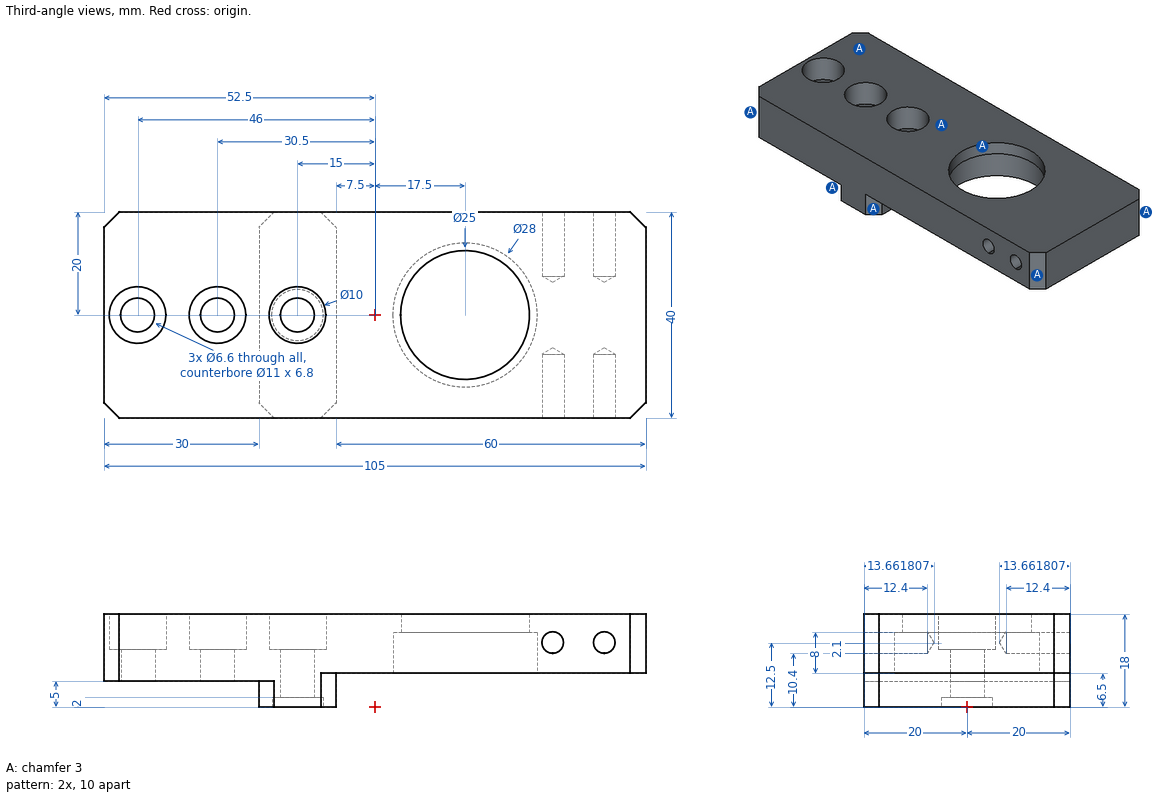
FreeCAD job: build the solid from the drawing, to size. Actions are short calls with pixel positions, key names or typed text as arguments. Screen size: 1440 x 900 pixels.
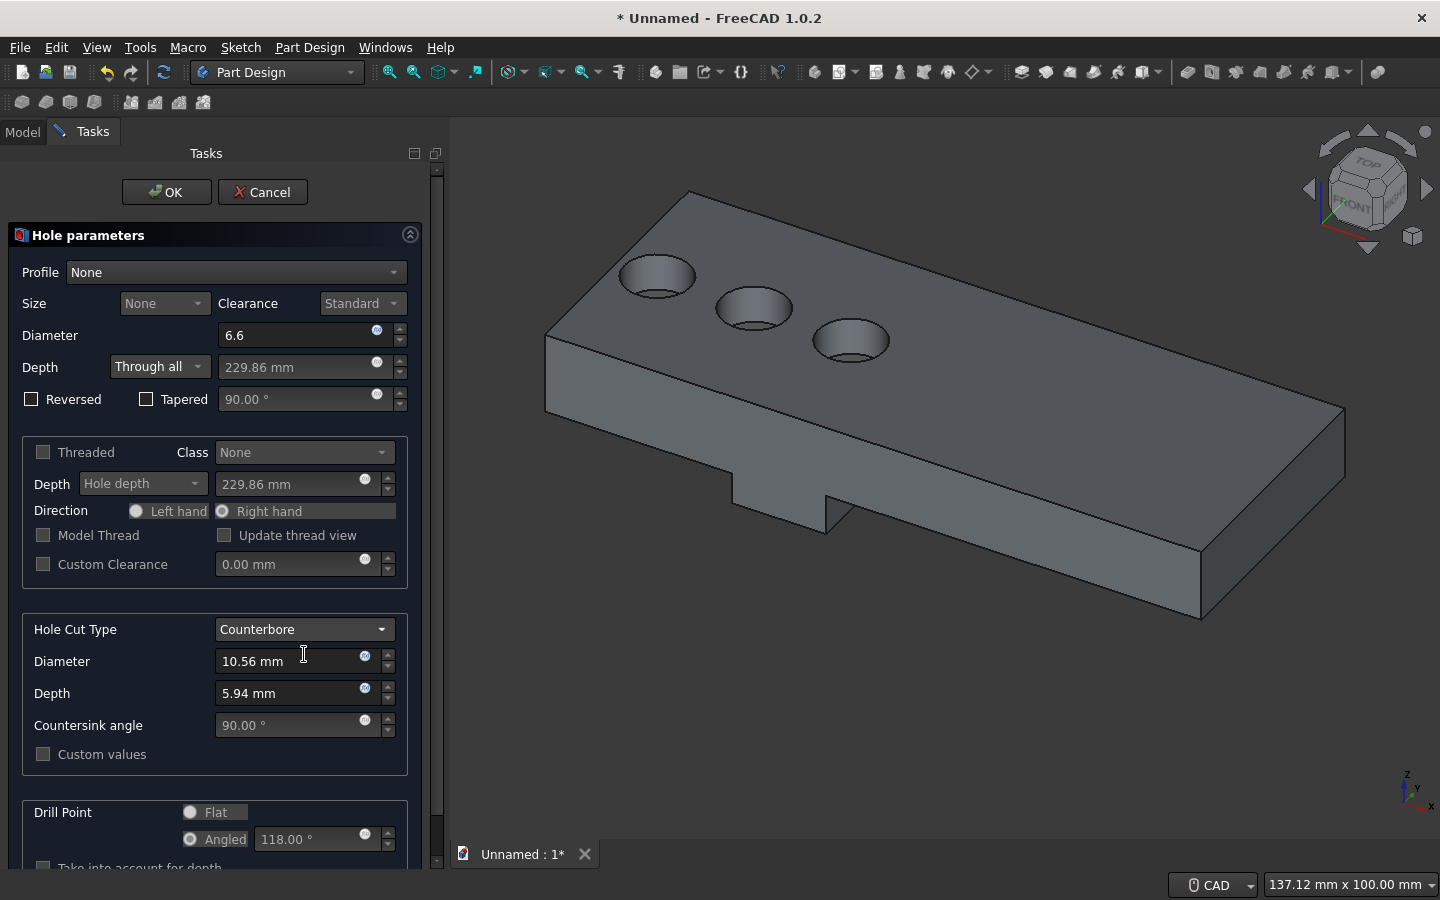
triple_click(298, 661)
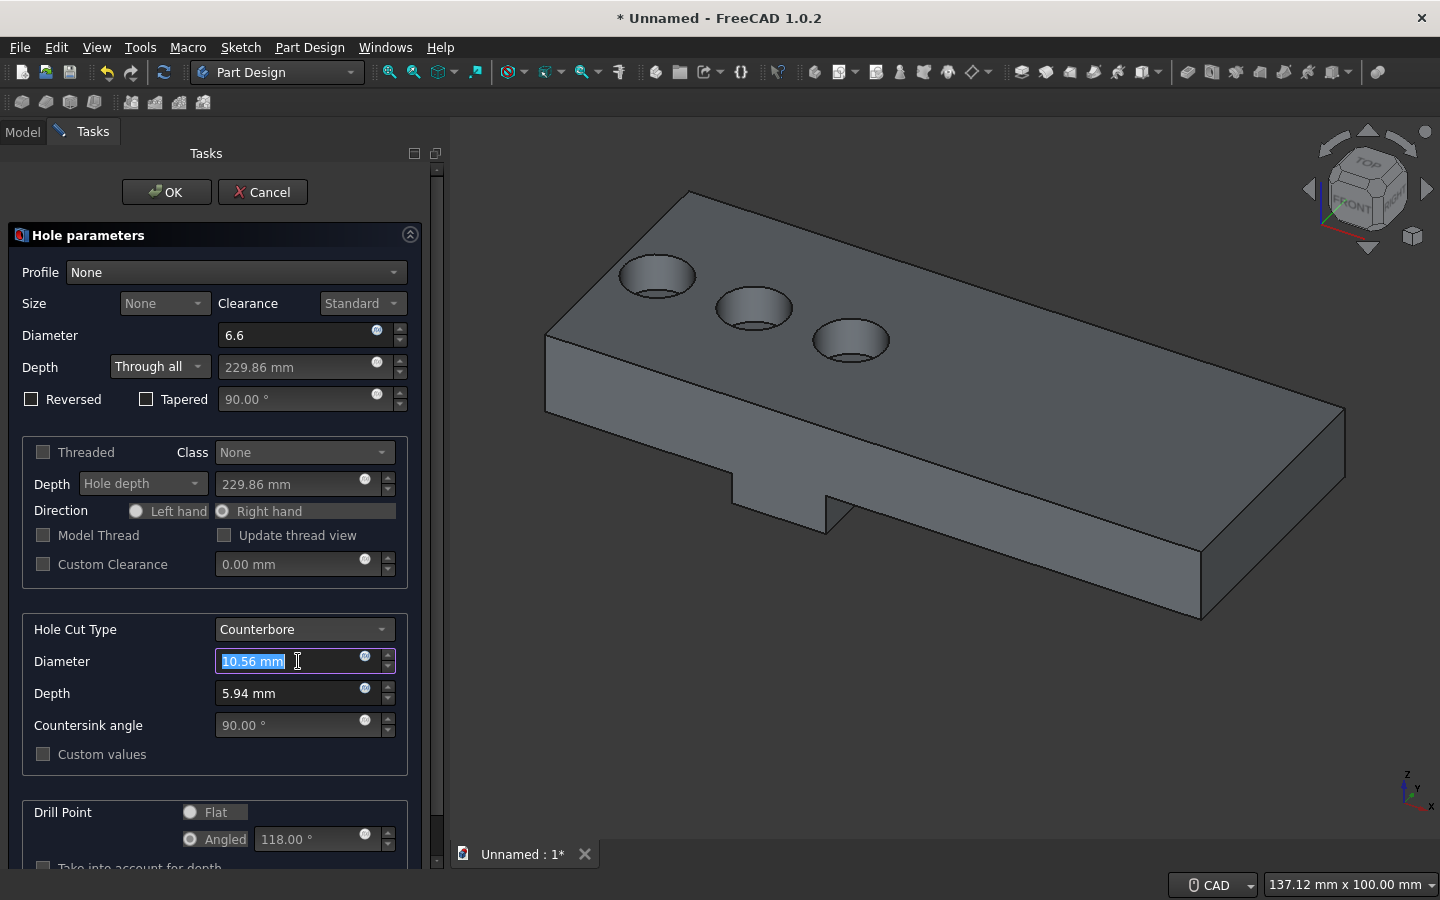
text(11)
key(Tab)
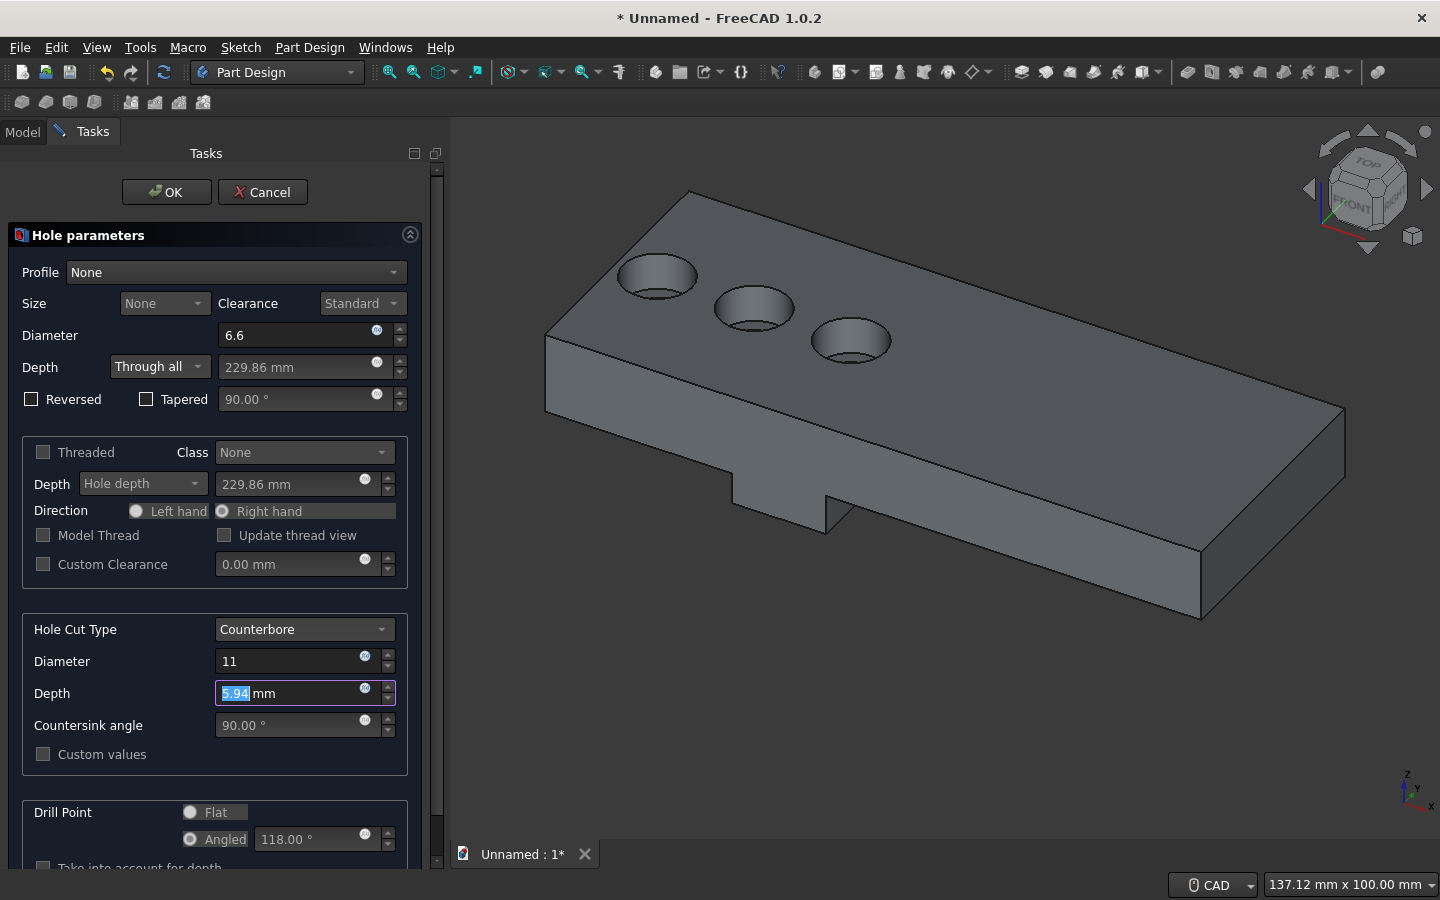
text(6.8)
key(Tab)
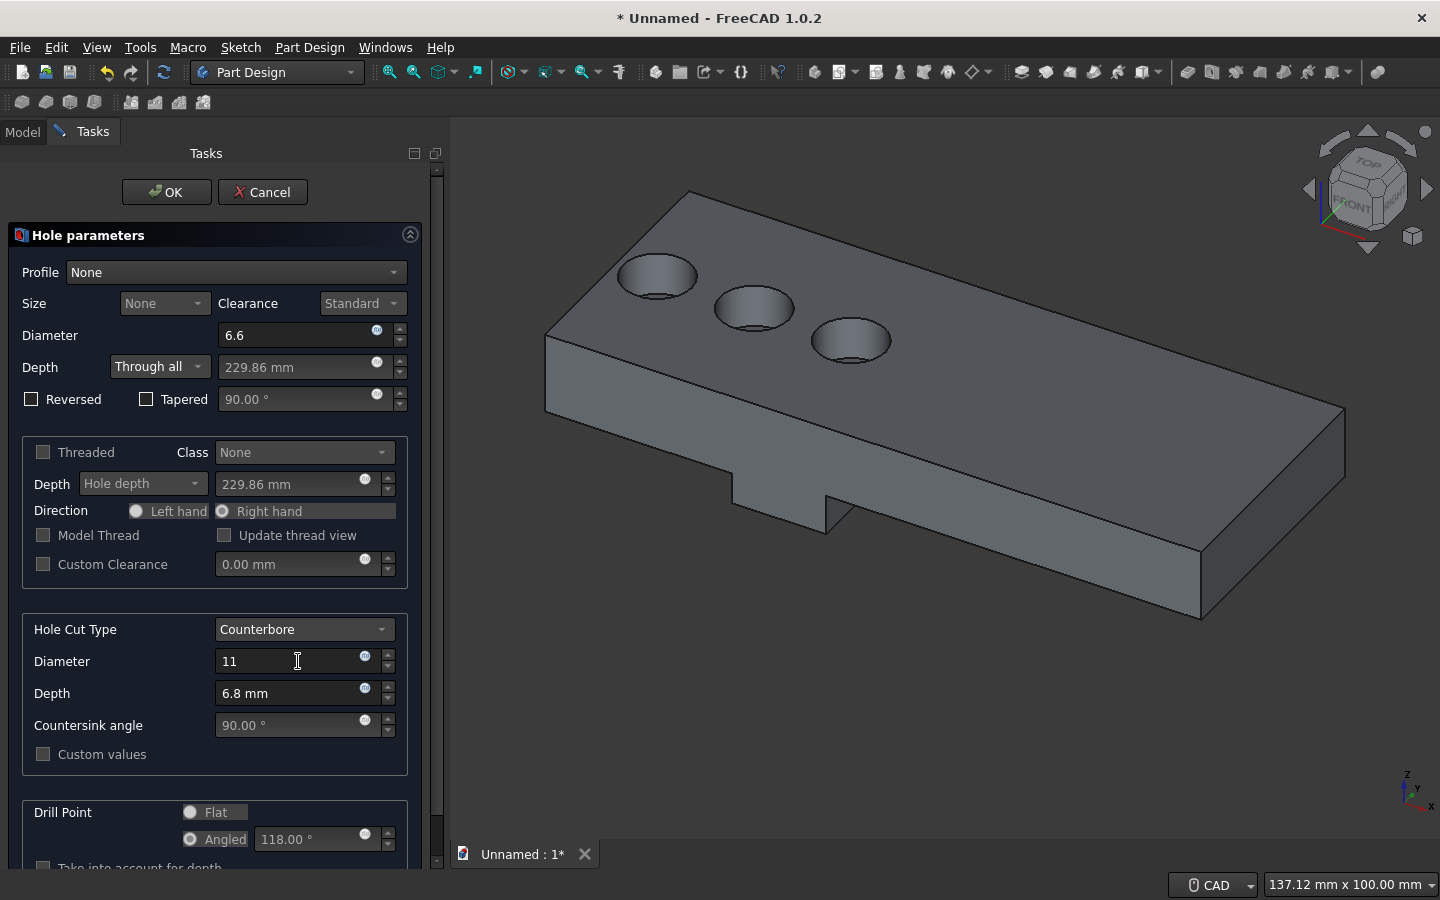
click(167, 192)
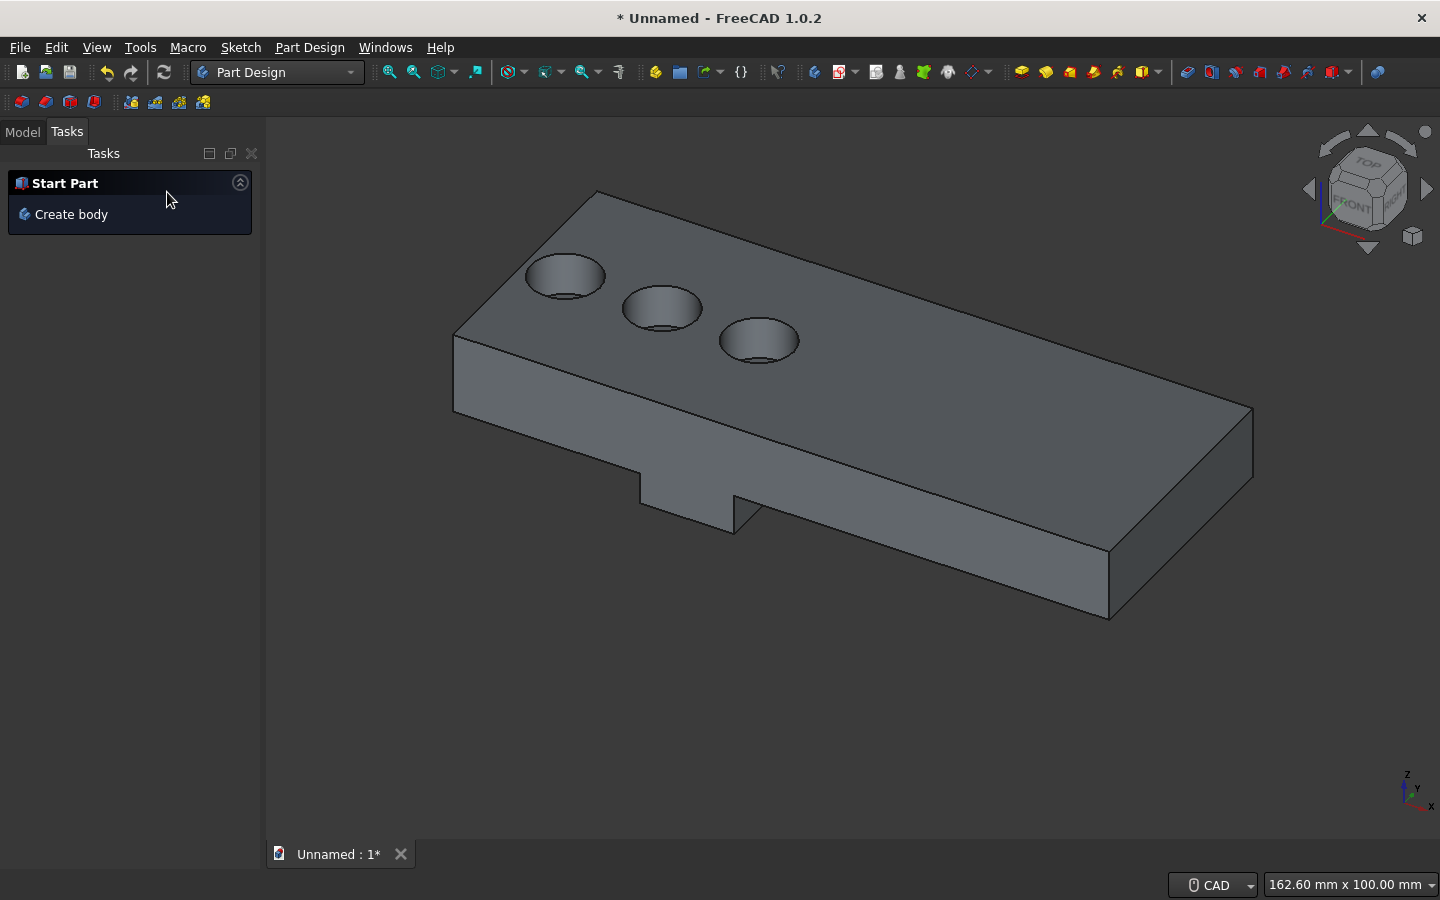
click(840, 72)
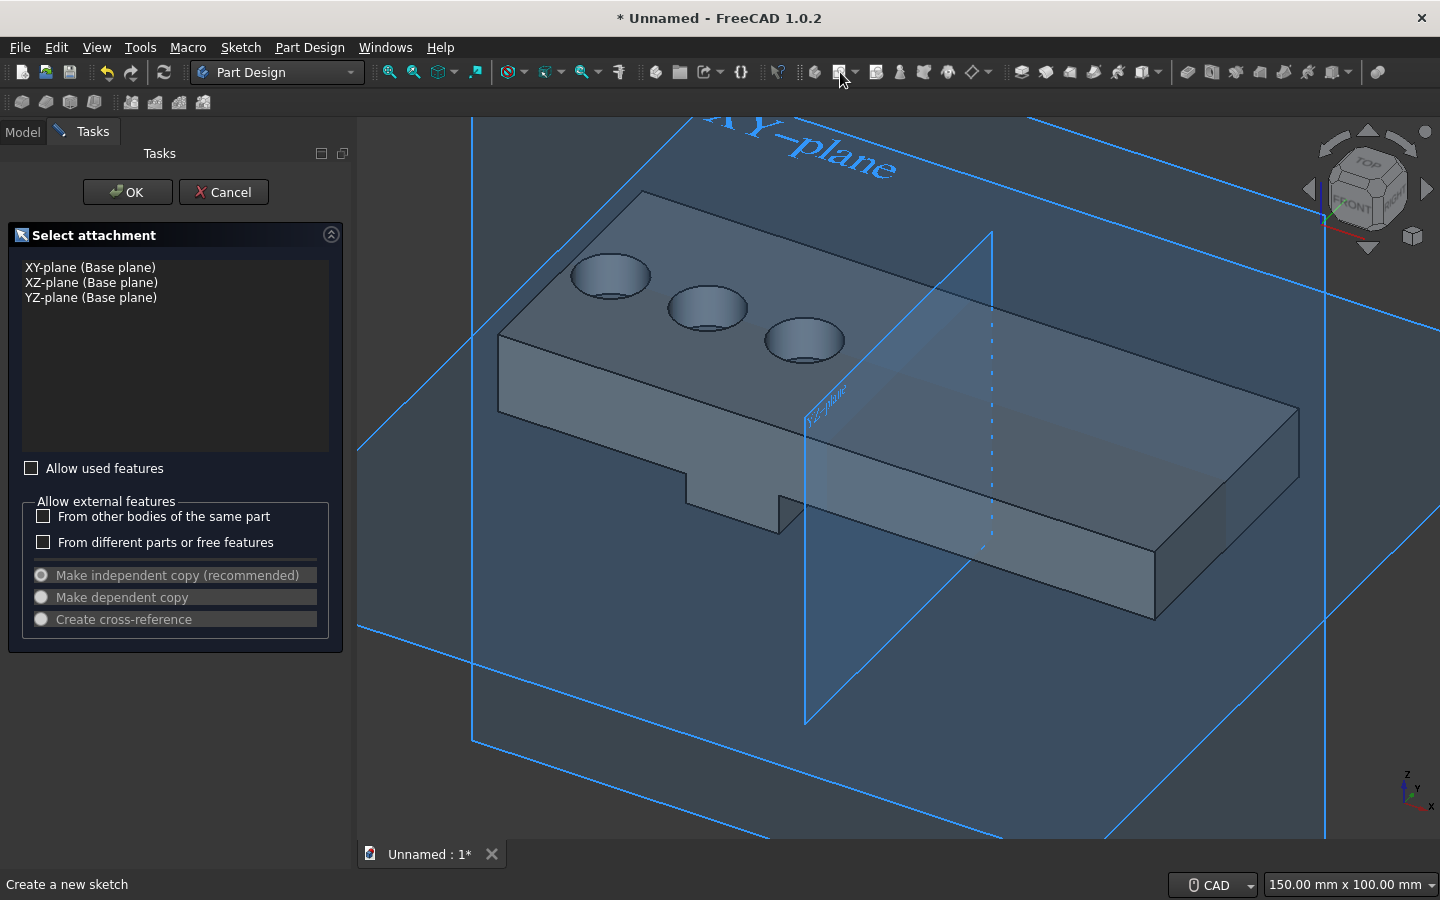
click(82, 268)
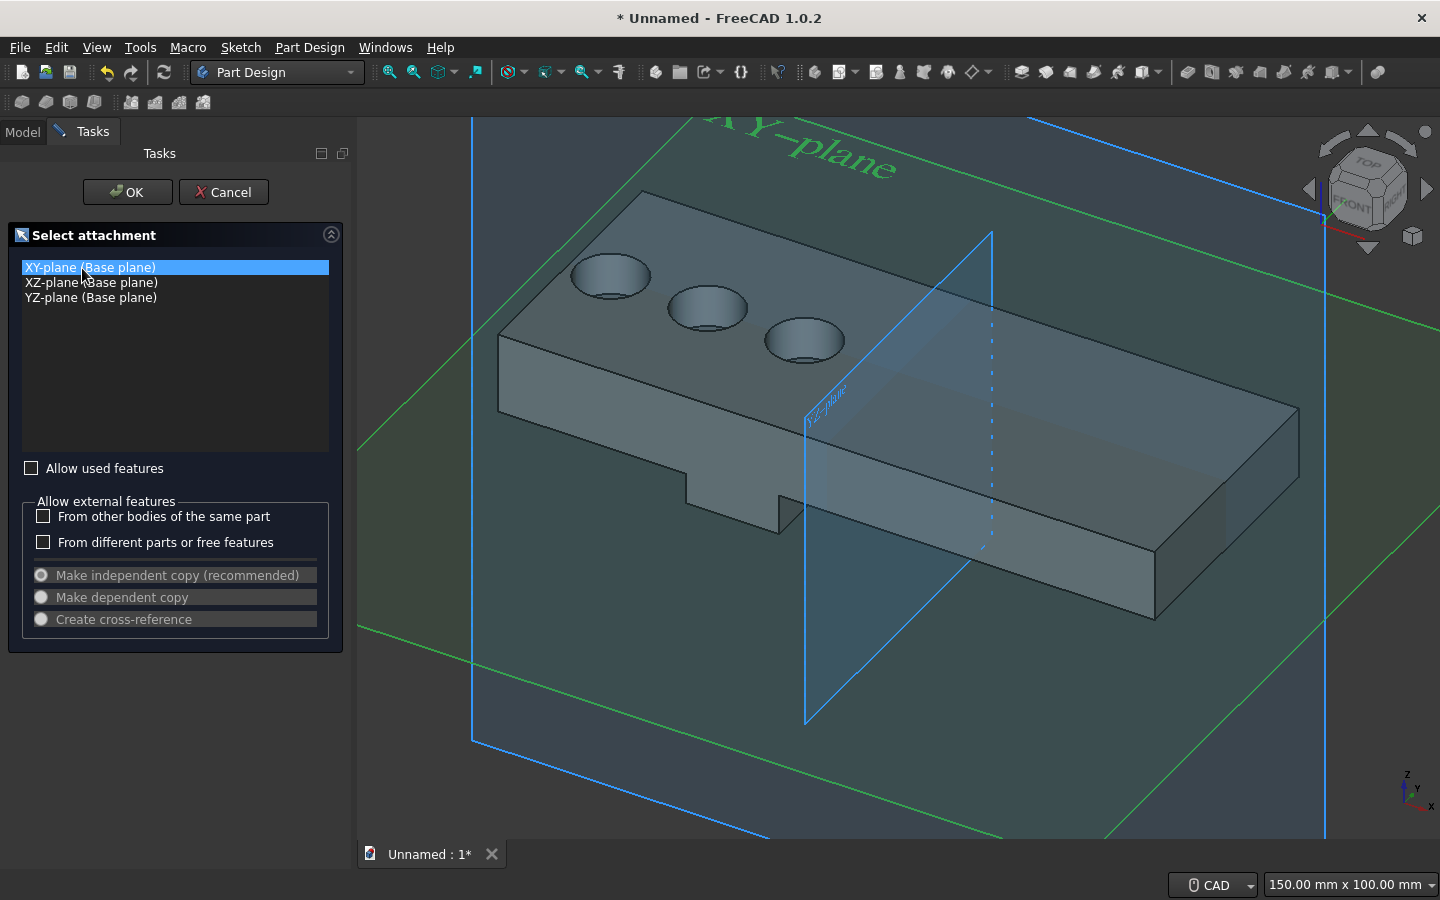
click(128, 192)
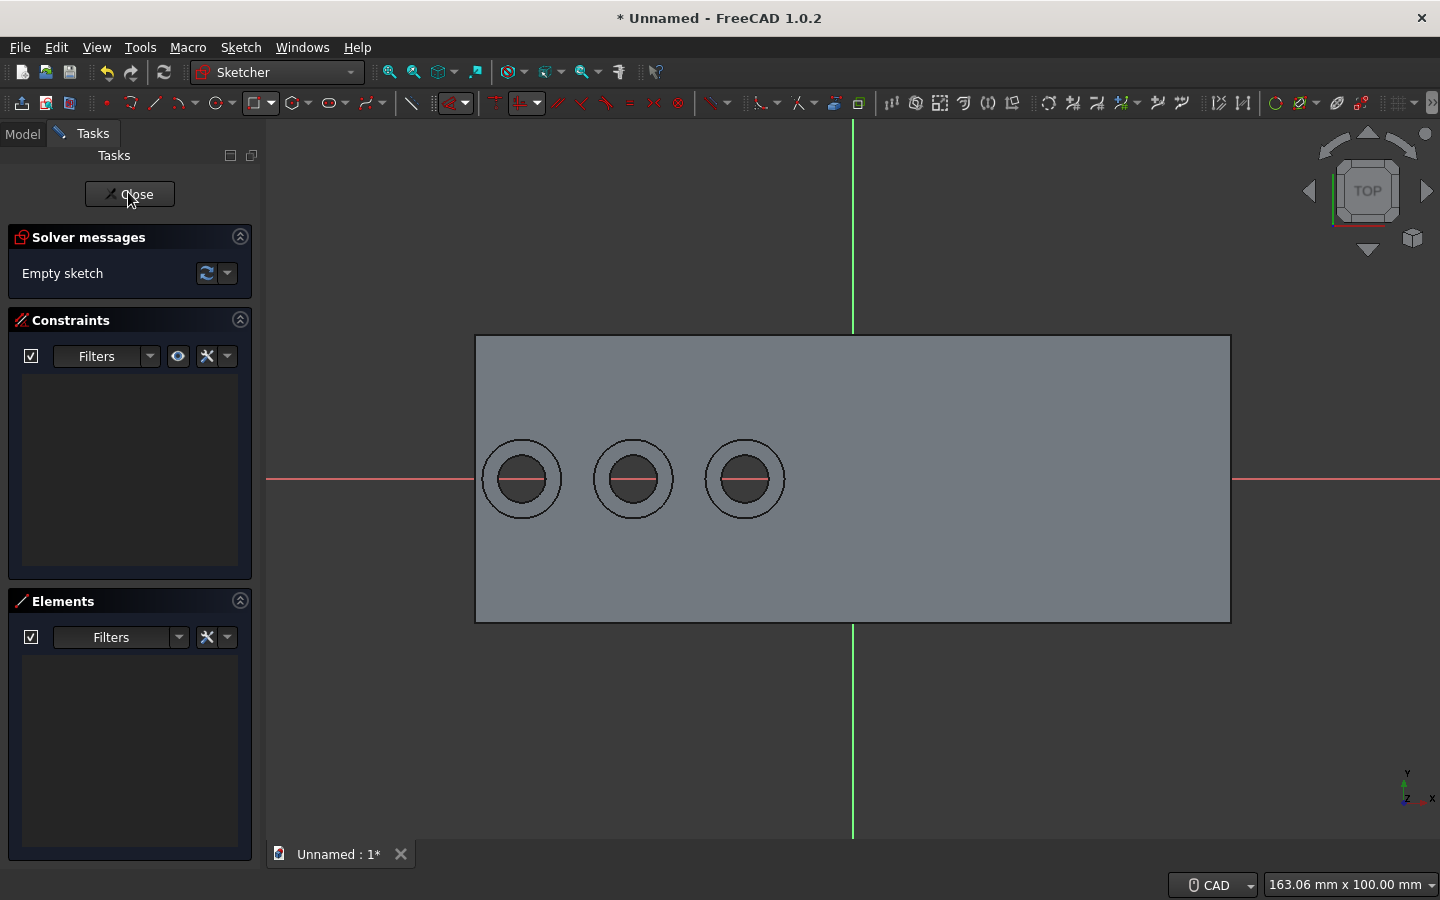
click(70, 104)